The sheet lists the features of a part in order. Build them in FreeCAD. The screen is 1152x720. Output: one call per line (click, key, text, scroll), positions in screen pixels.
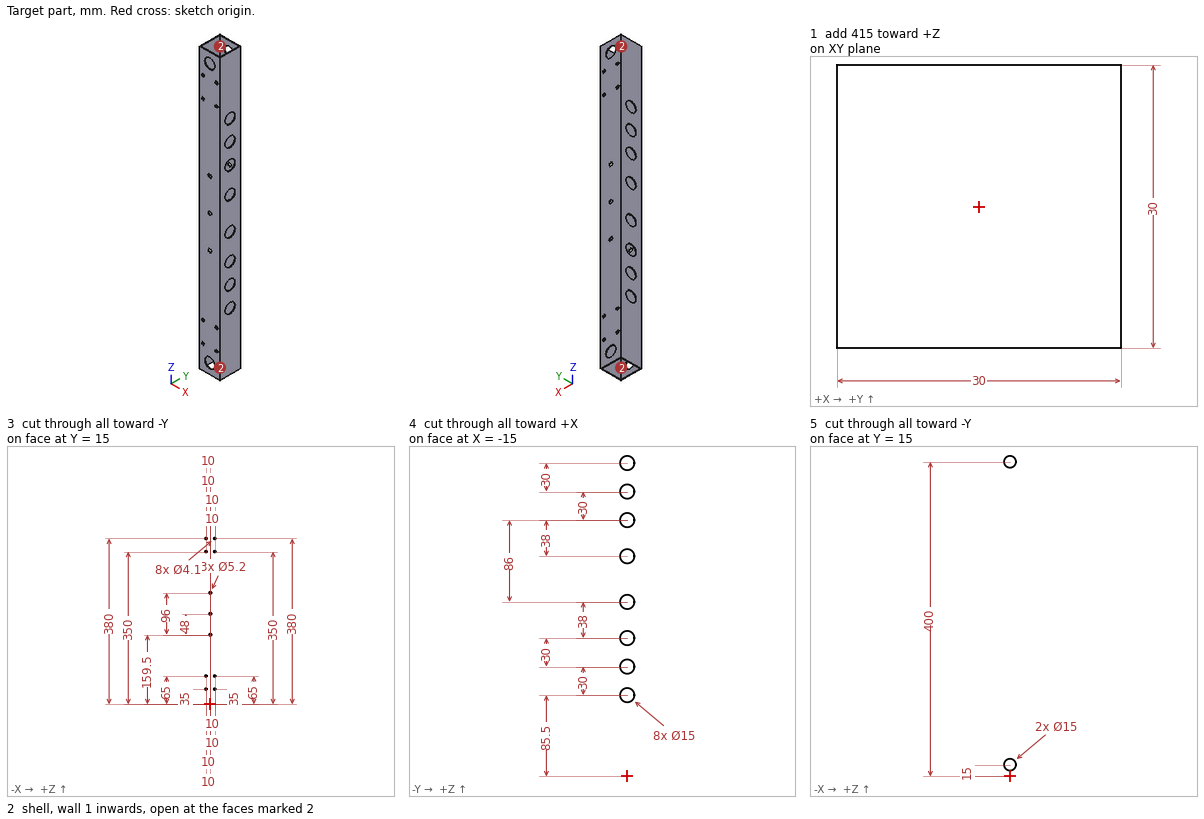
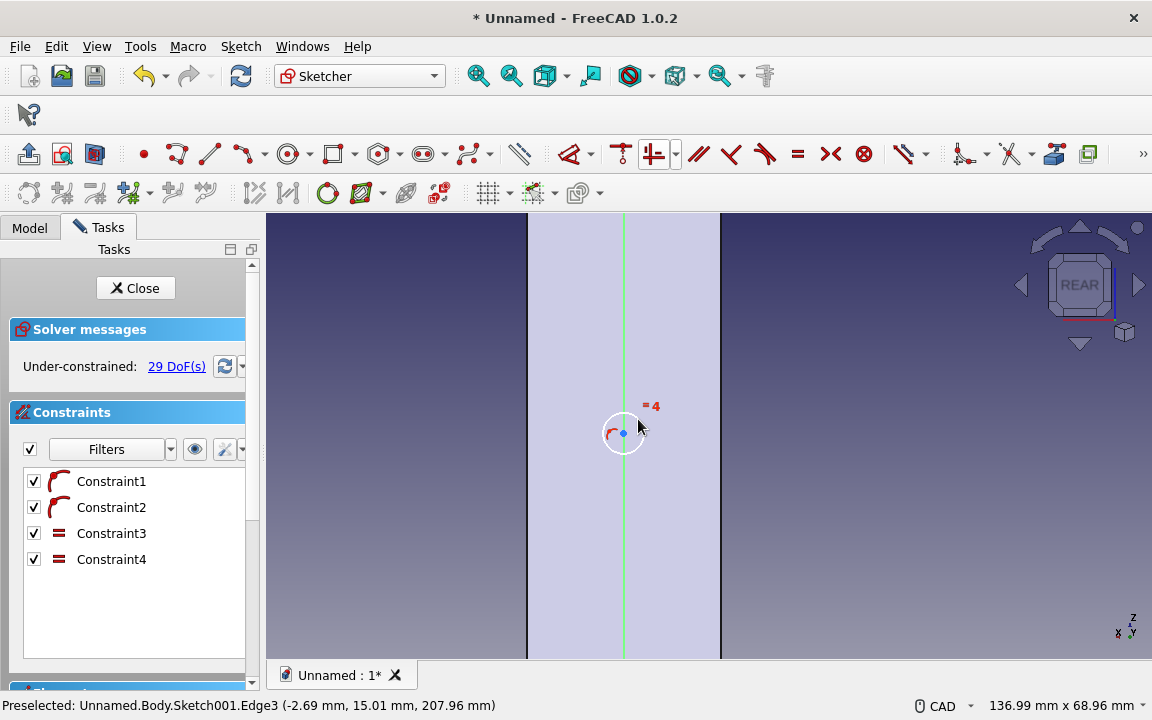
scroll(643, 424, down, 11)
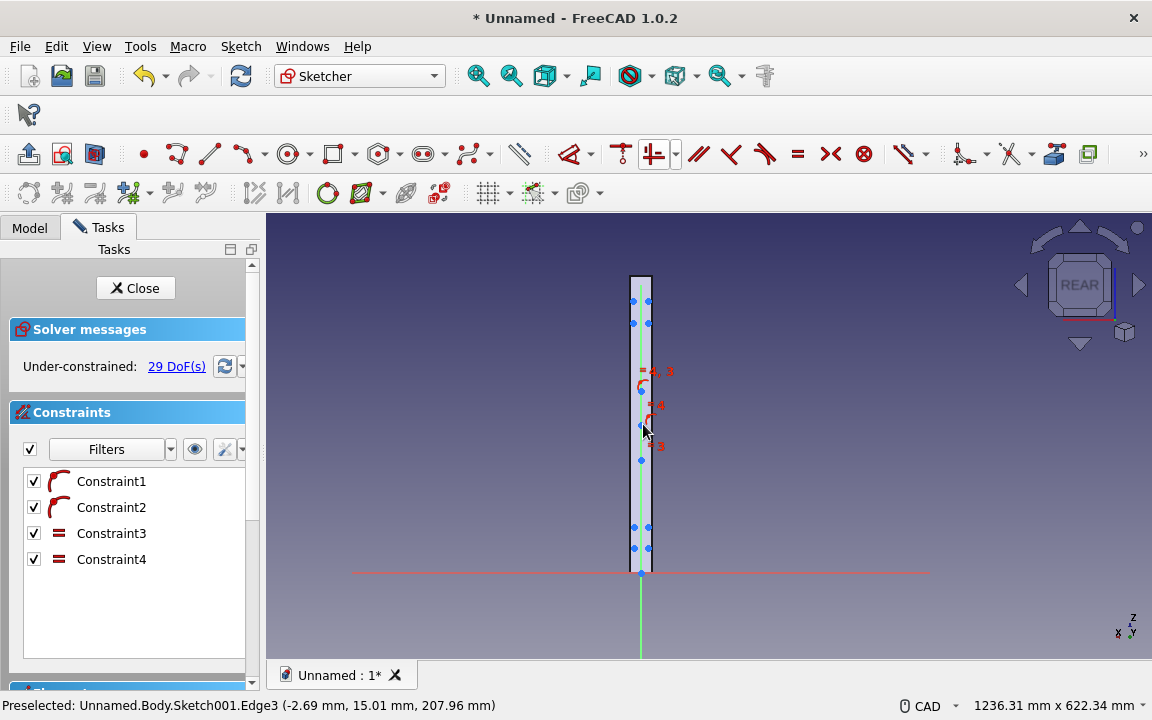
scroll(650, 548, up, 11)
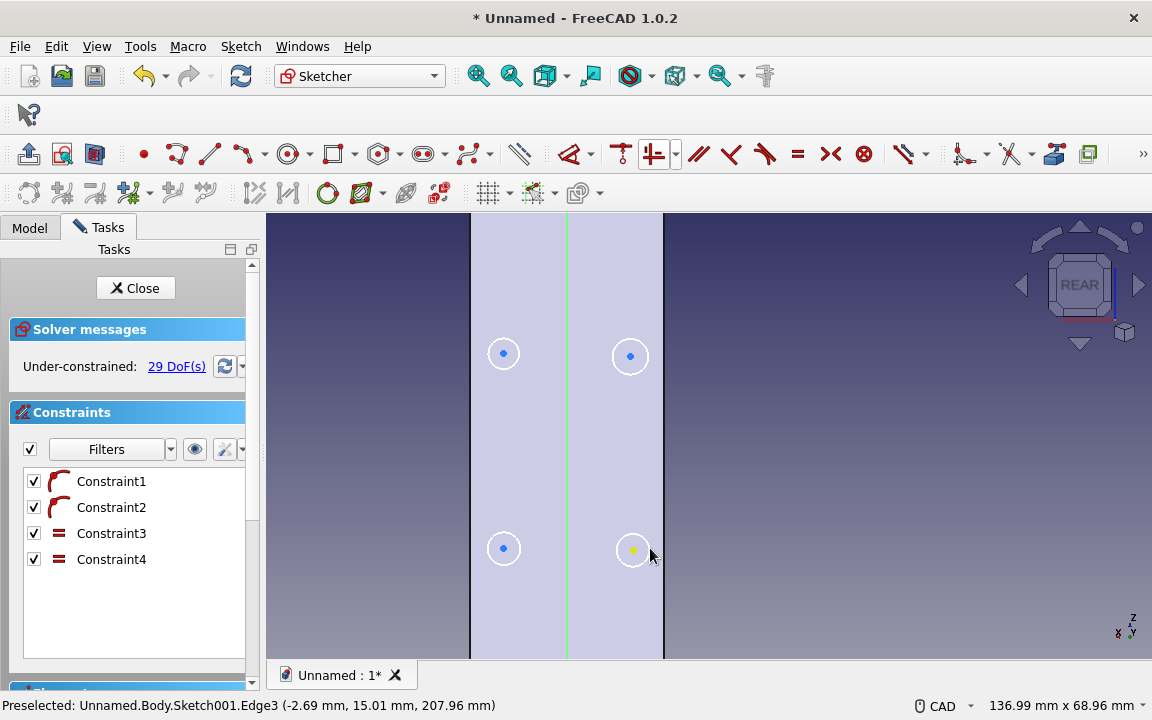
click(645, 539)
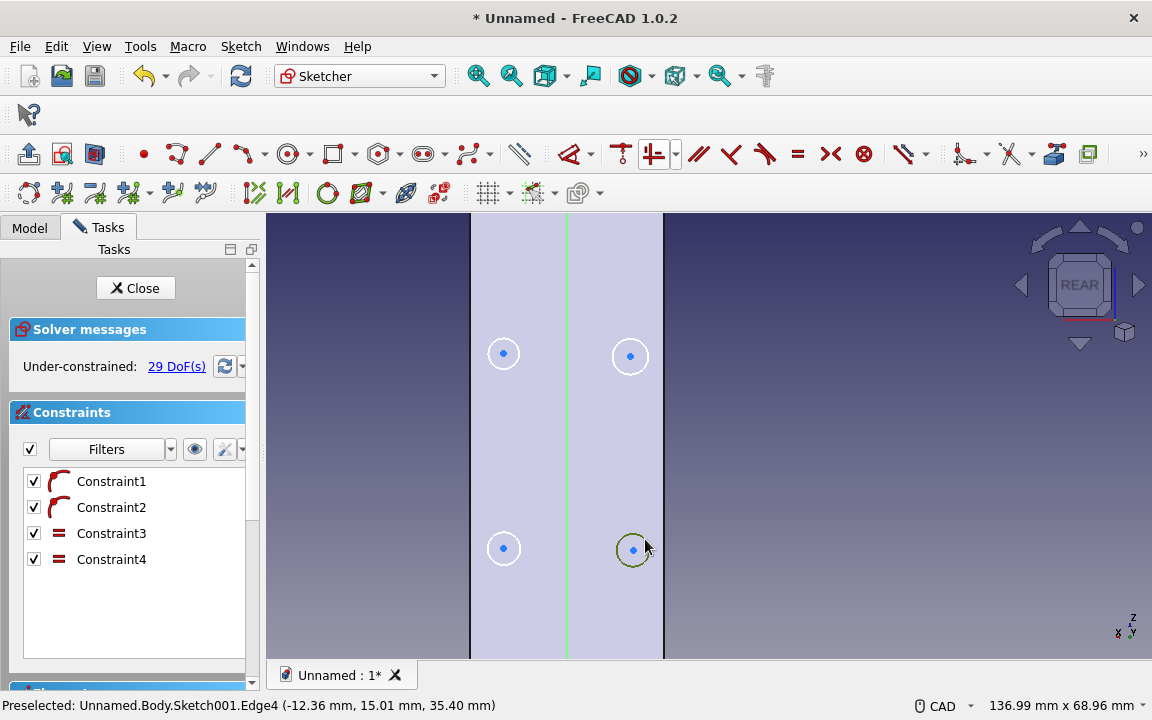
scroll(650, 548, down, 11)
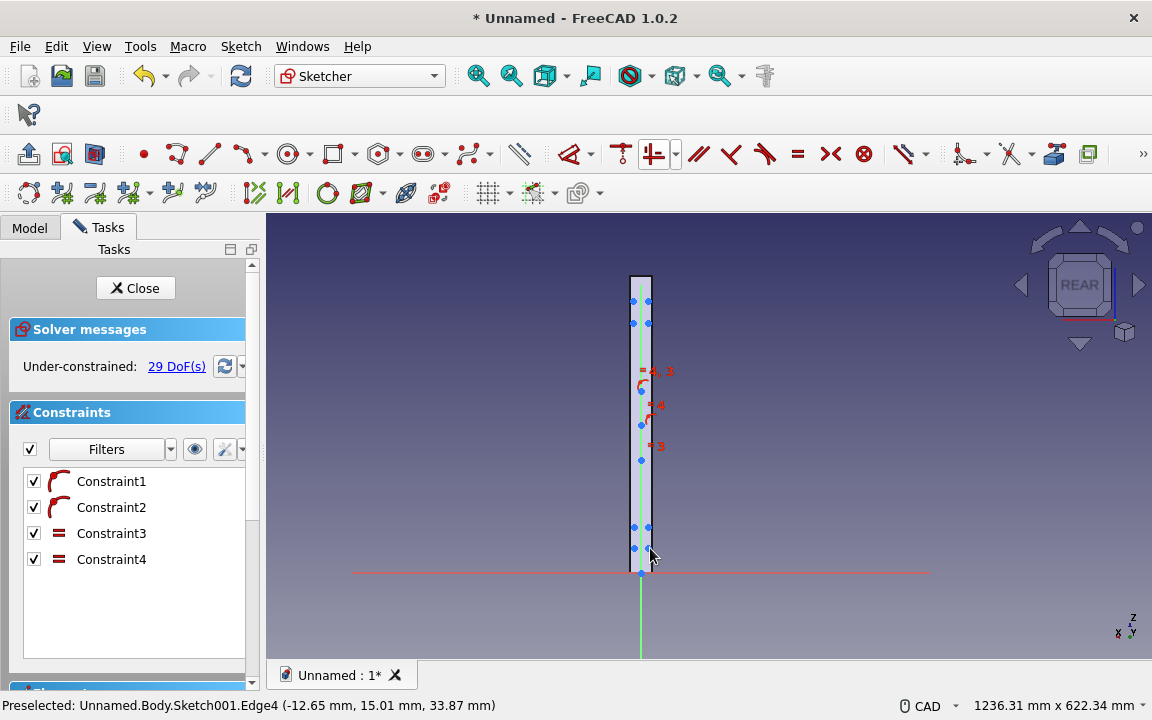
scroll(650, 300, up, 11)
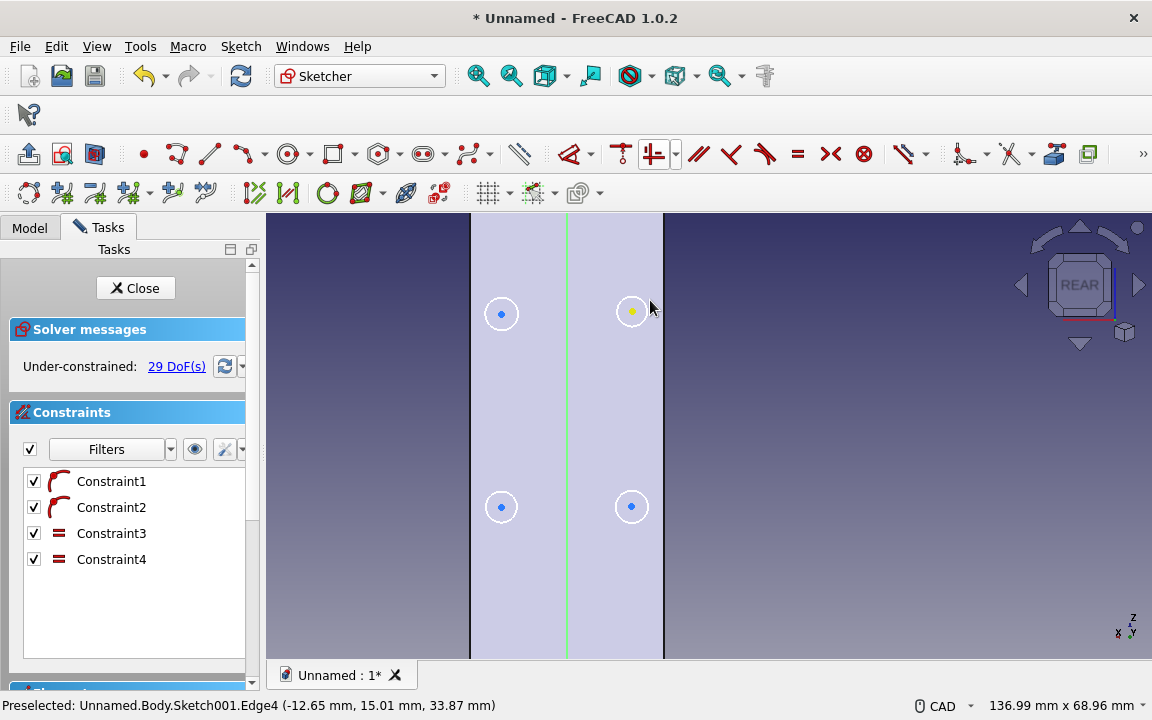
click(643, 301)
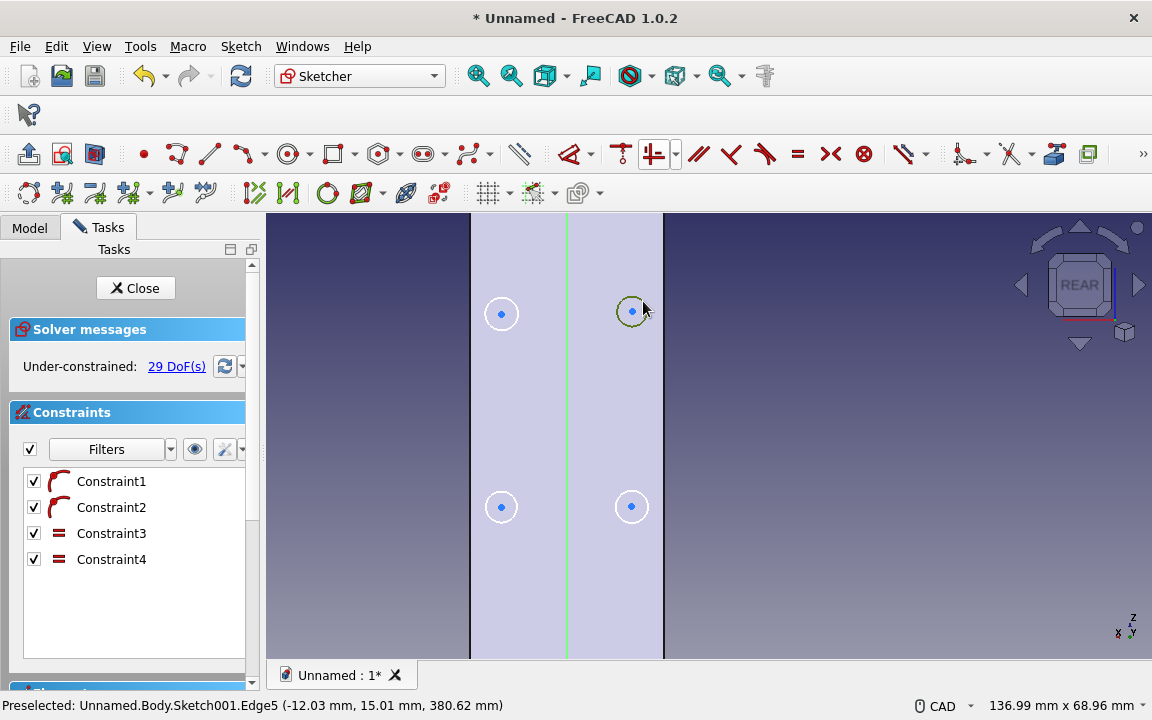
scroll(650, 300, down, 11)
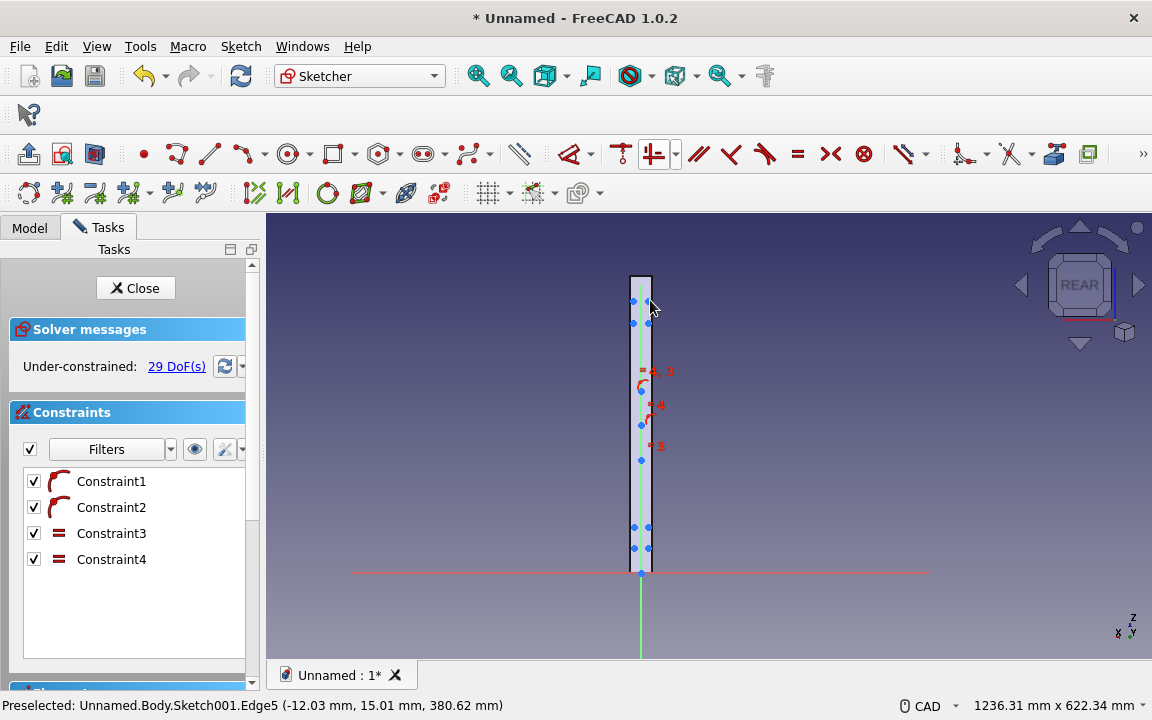
scroll(650, 526, up, 10)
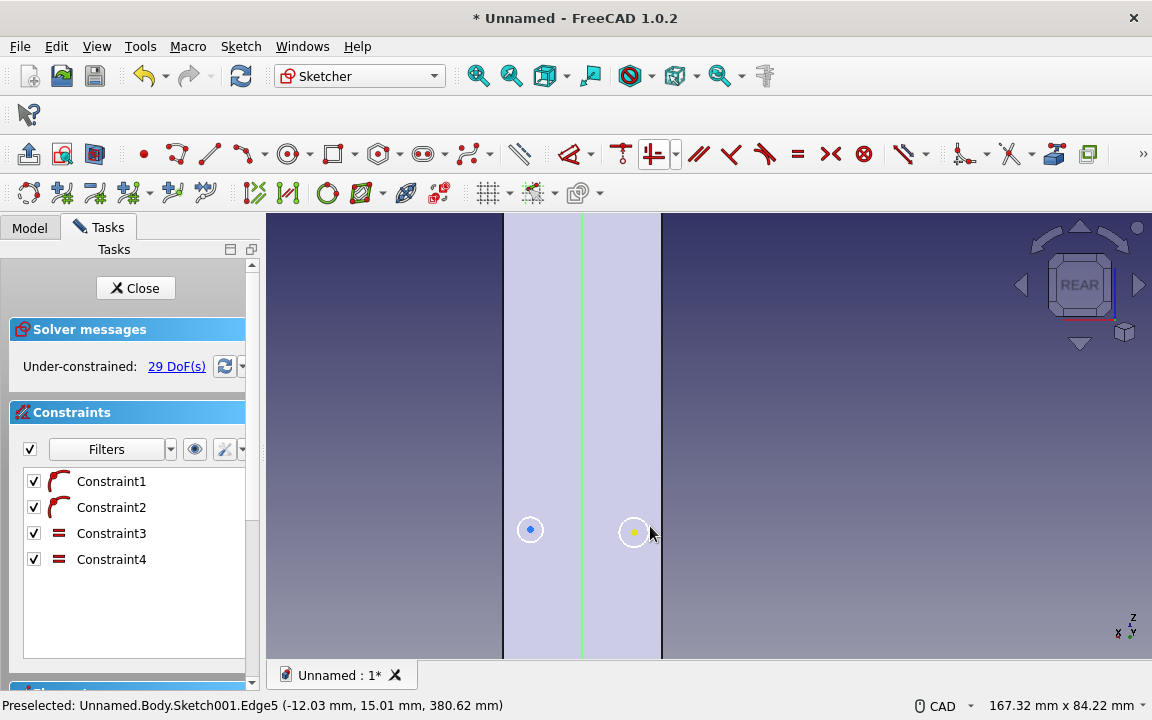
click(644, 522)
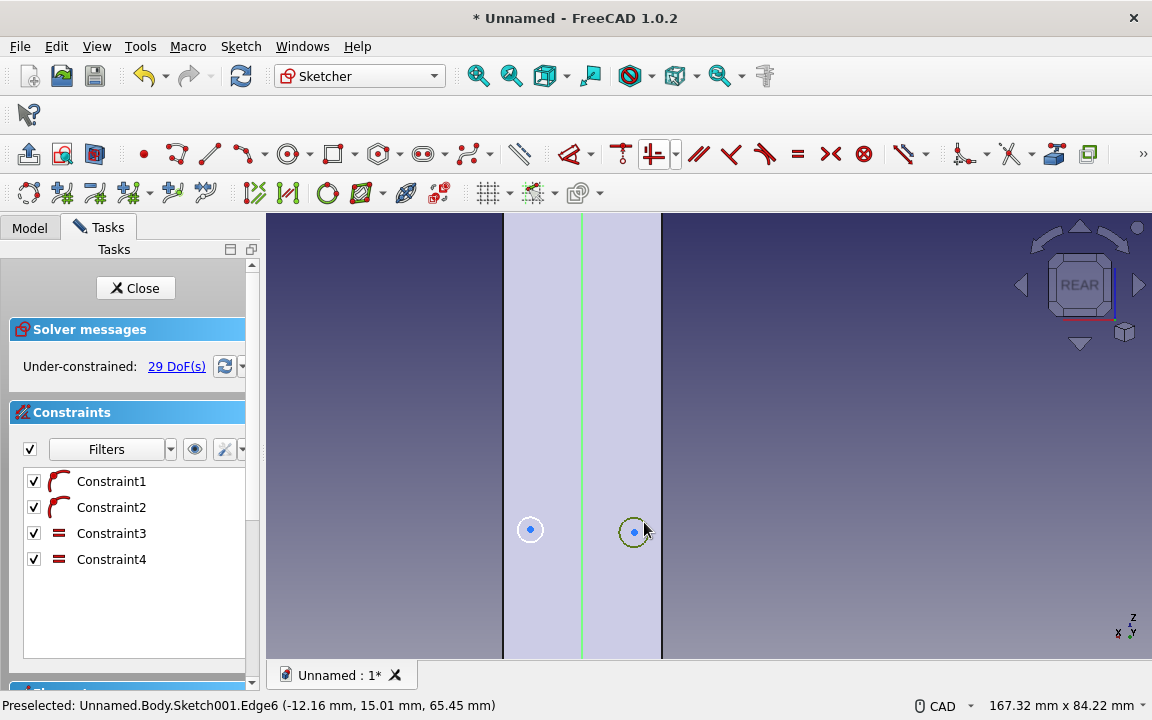
scroll(650, 526, down, 10)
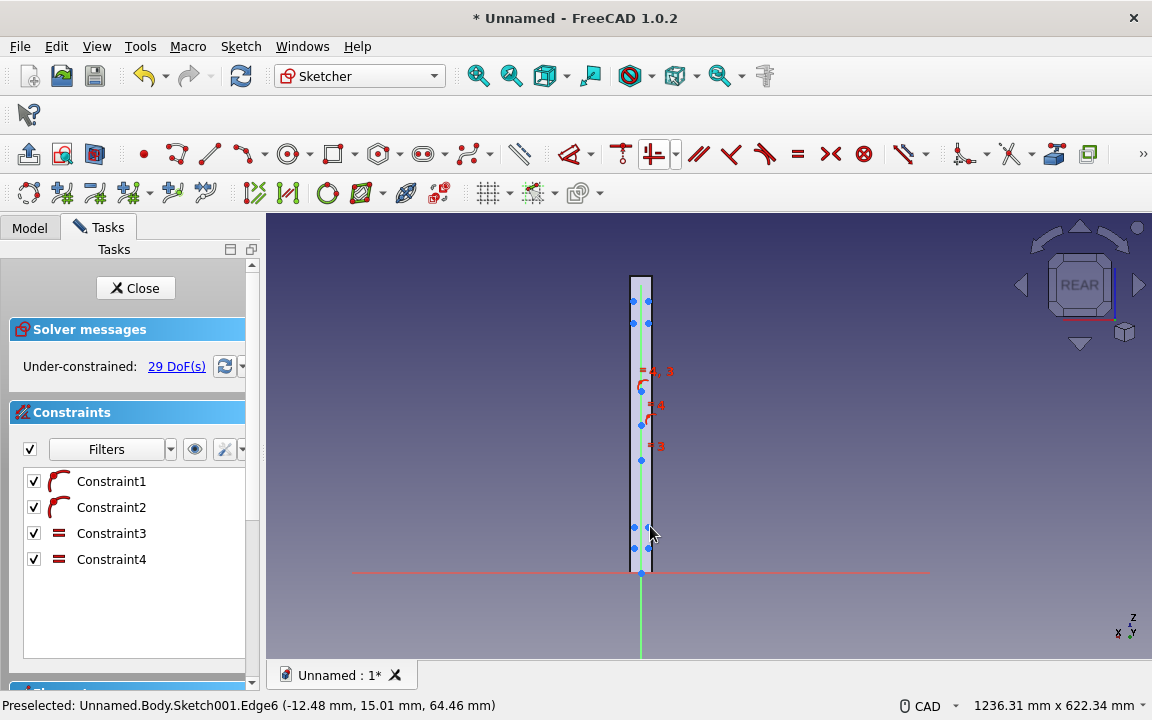
scroll(650, 322, up, 11)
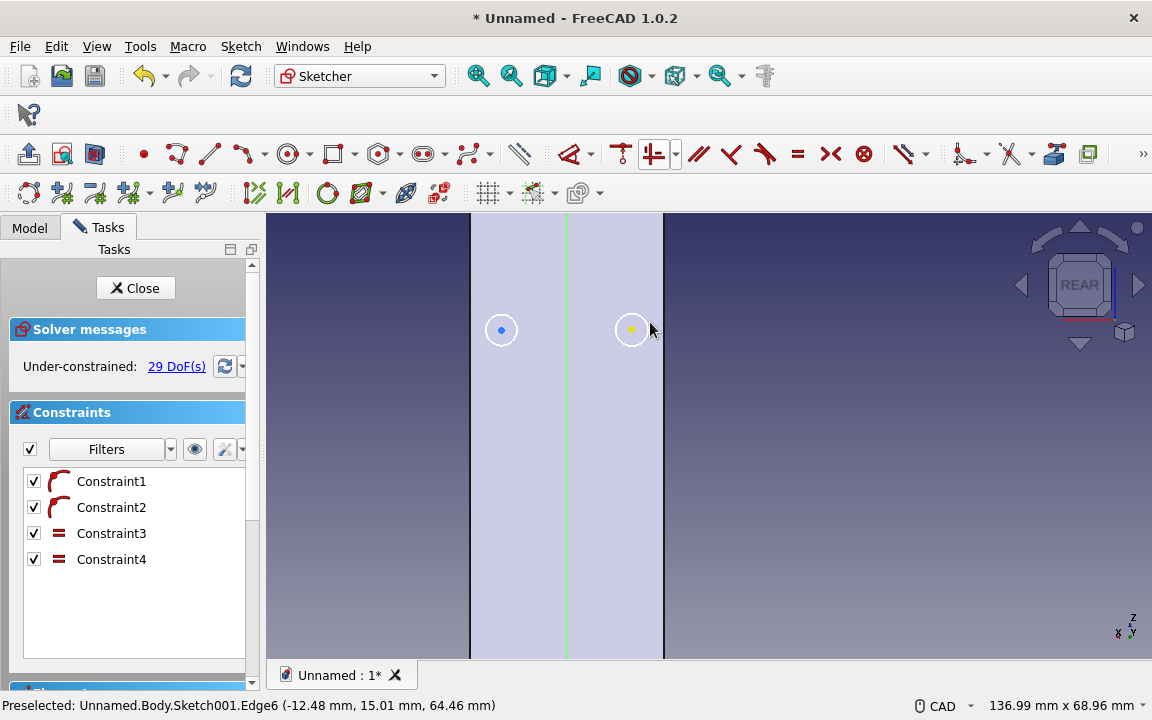
click(643, 318)